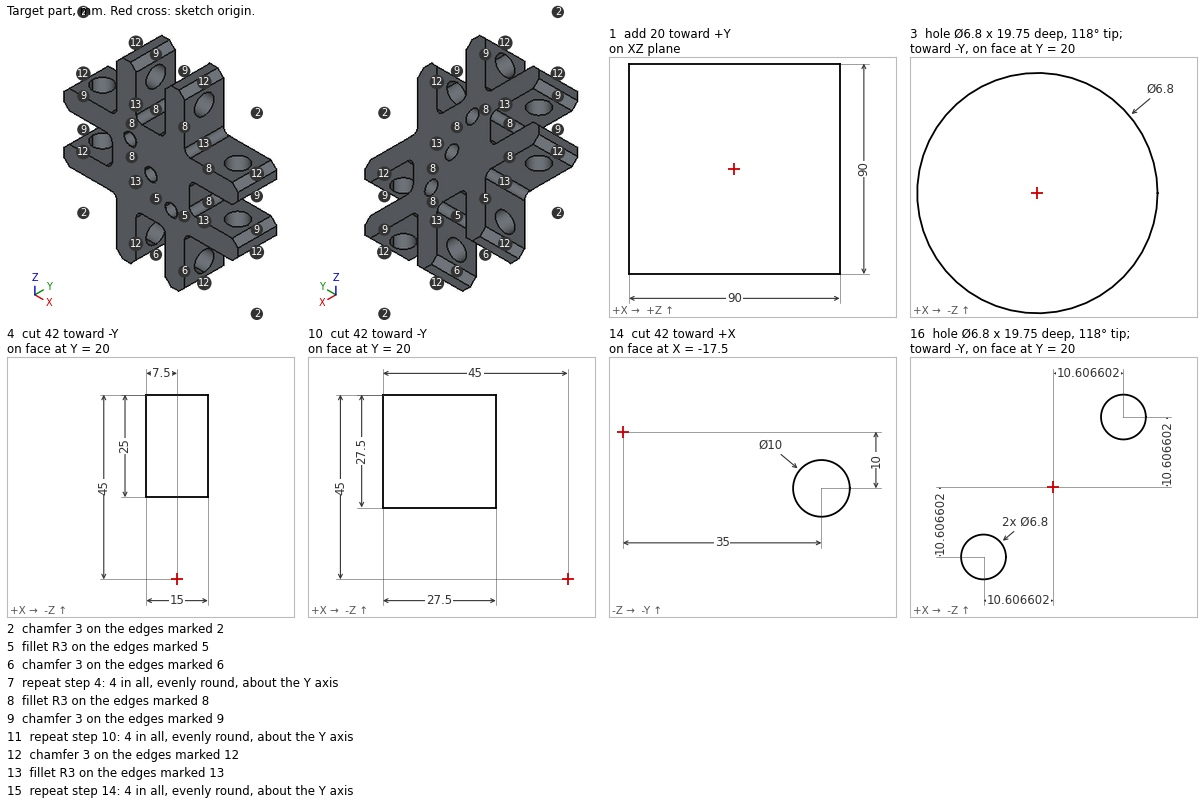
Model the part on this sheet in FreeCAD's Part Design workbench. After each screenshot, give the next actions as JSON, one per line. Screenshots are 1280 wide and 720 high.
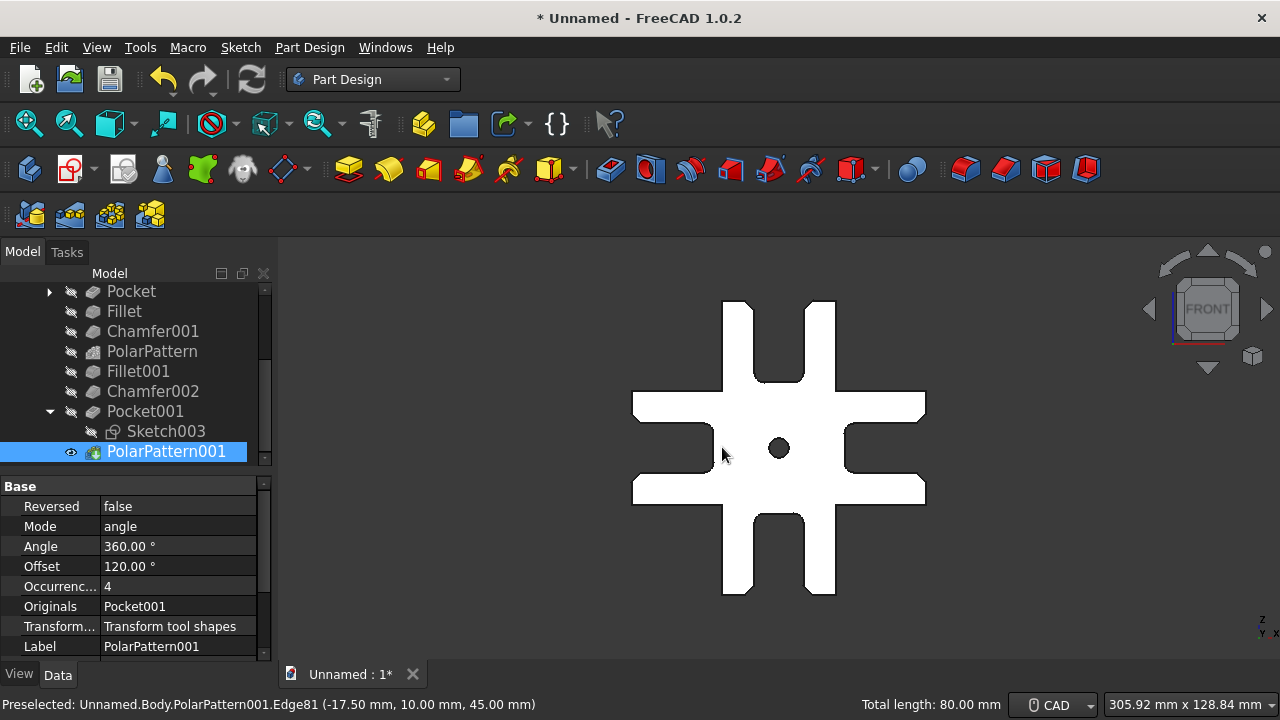
{"action": "key", "text": "3"}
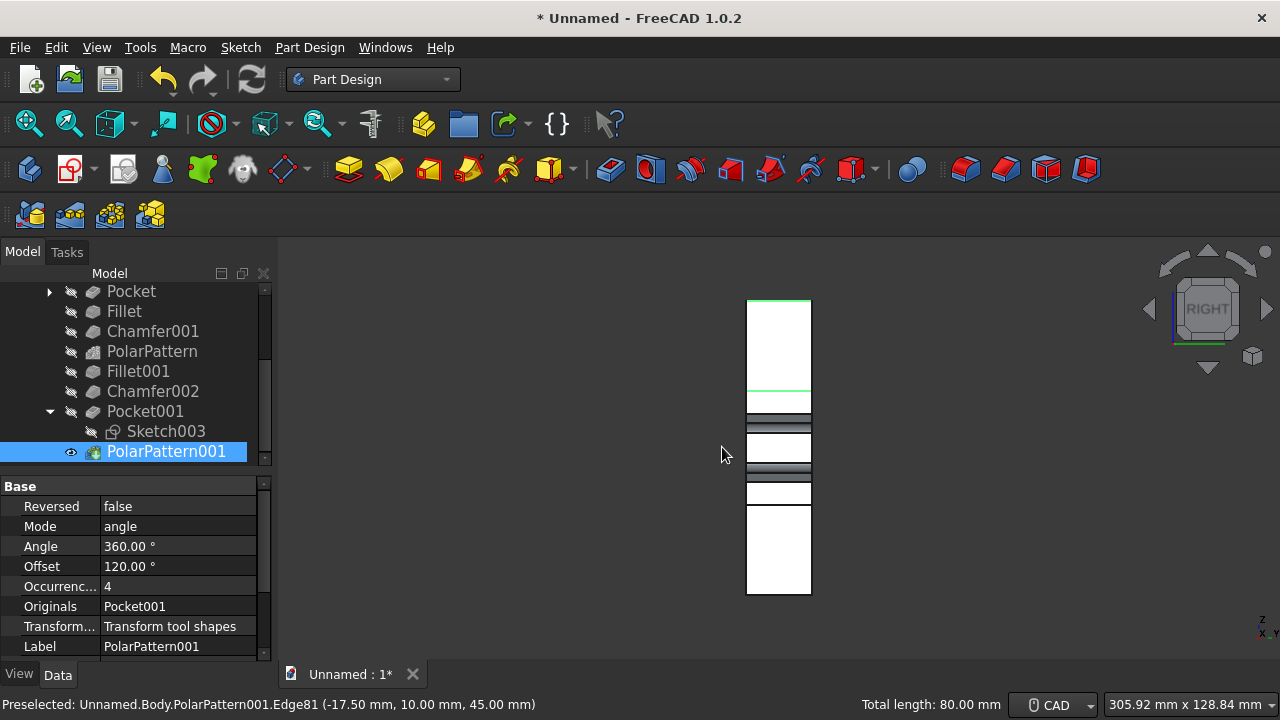
{"action": "left_click", "coordinate": [779, 504], "text": "ctrl"}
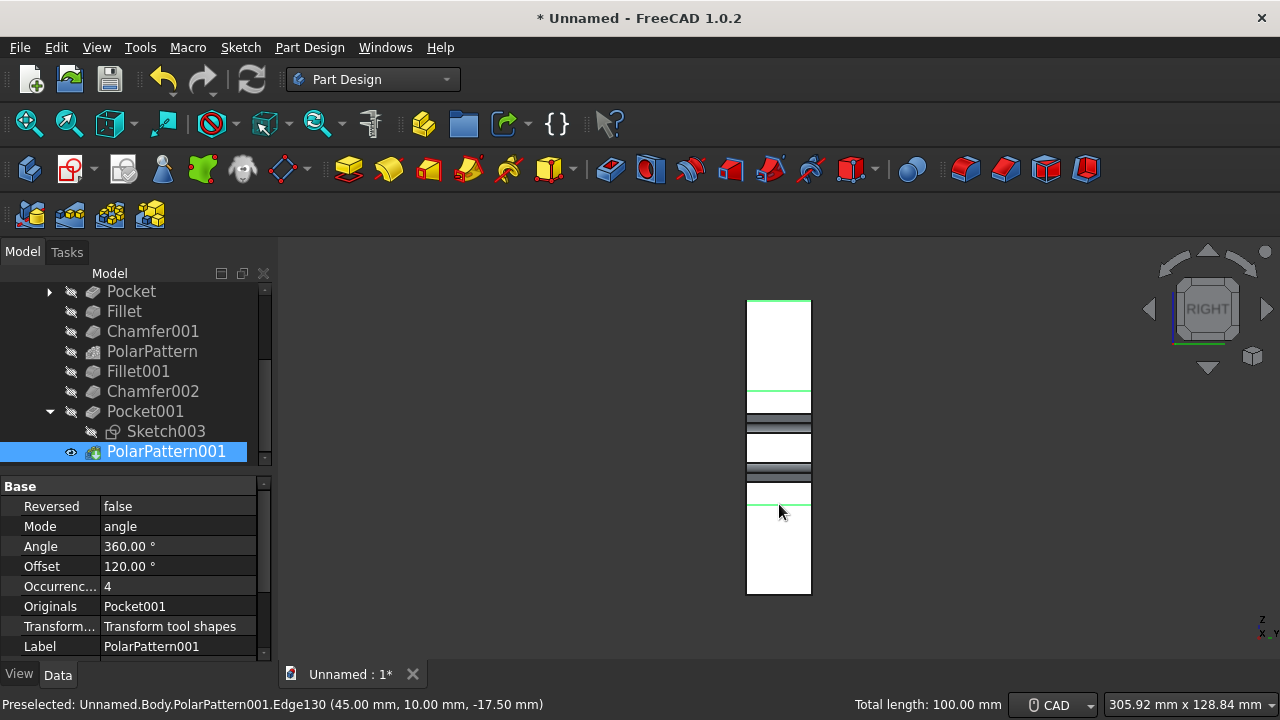
{"action": "left_click", "coordinate": [779, 594], "text": "ctrl"}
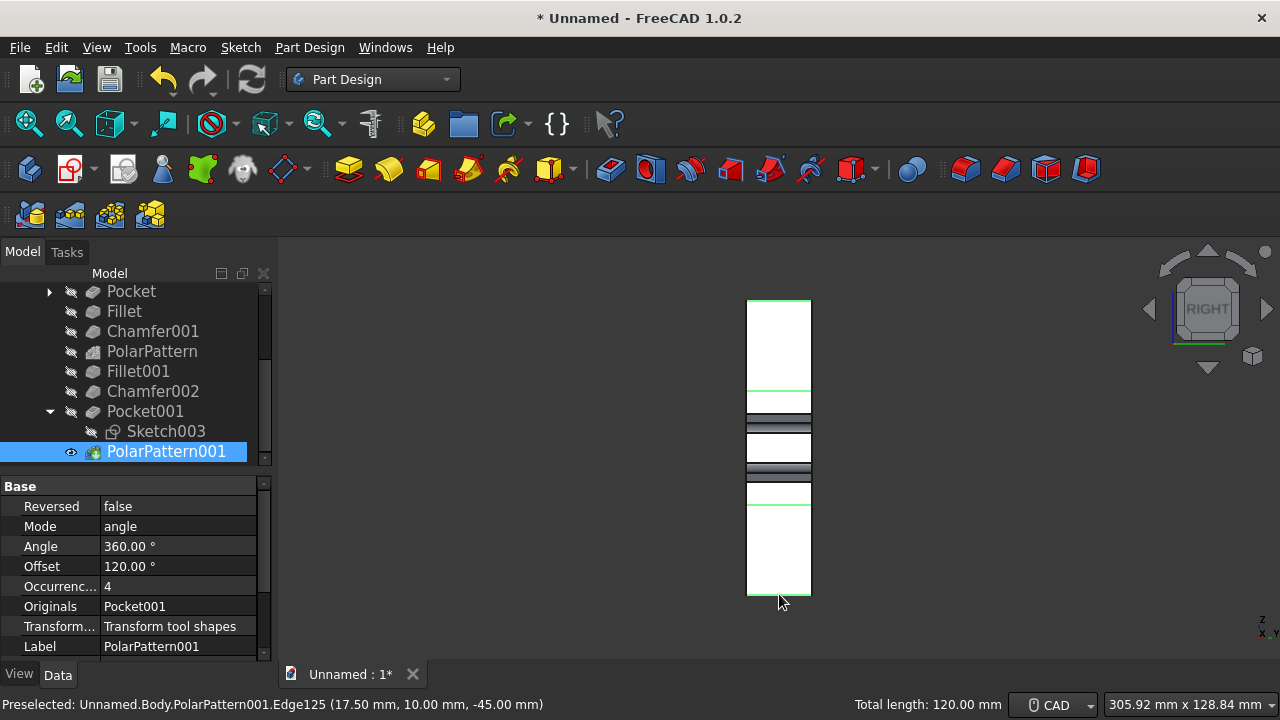
{"action": "key", "text": "5"}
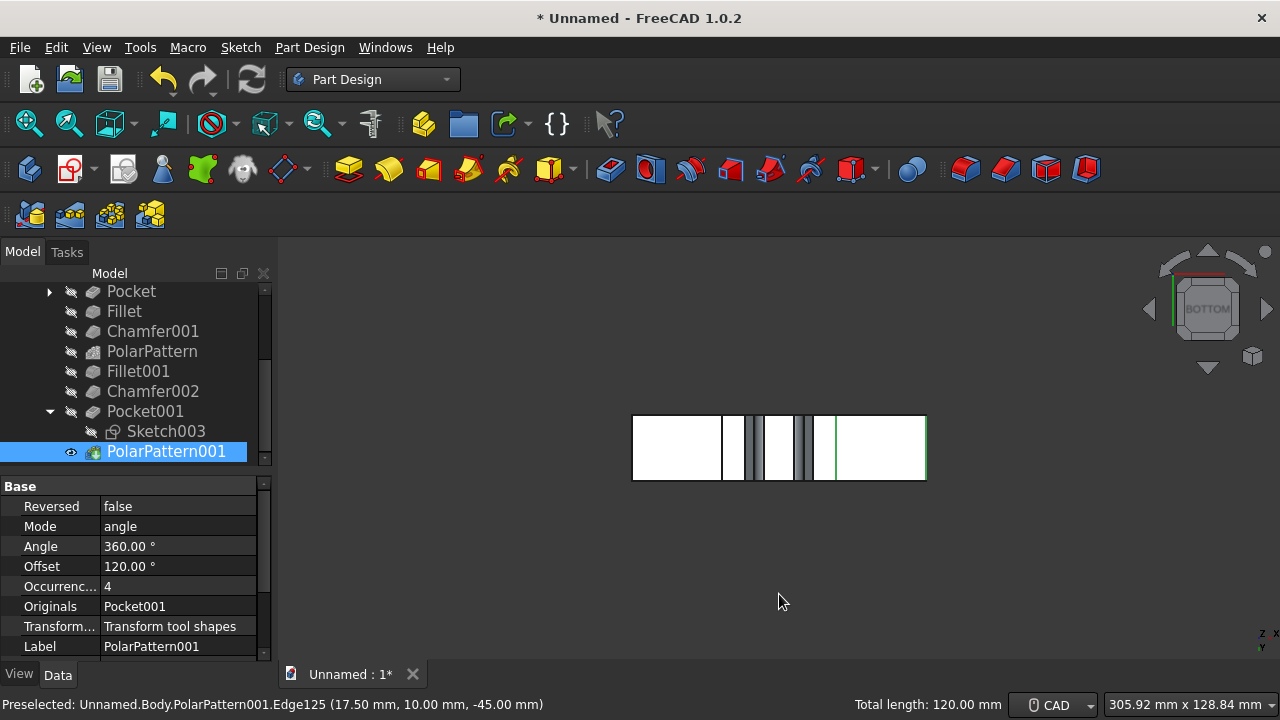
{"action": "left_click", "coordinate": [30, 124]}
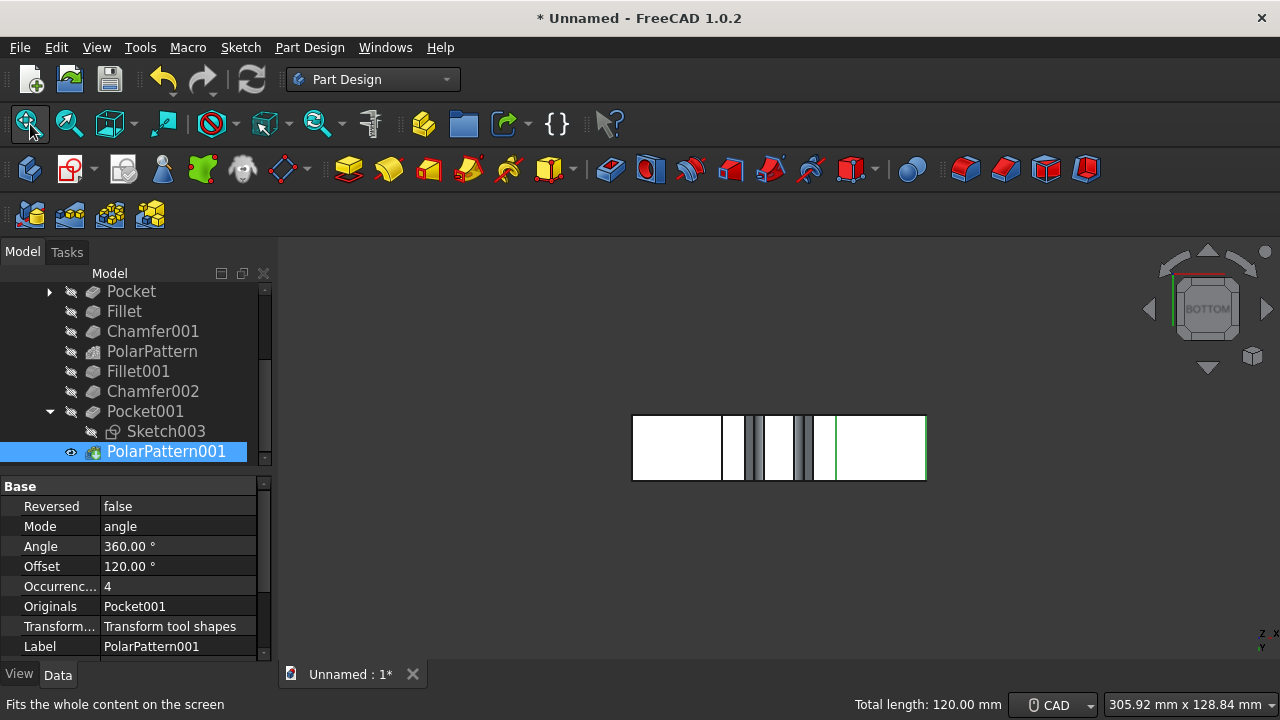
{"action": "left_click", "coordinate": [722, 447], "text": "ctrl"}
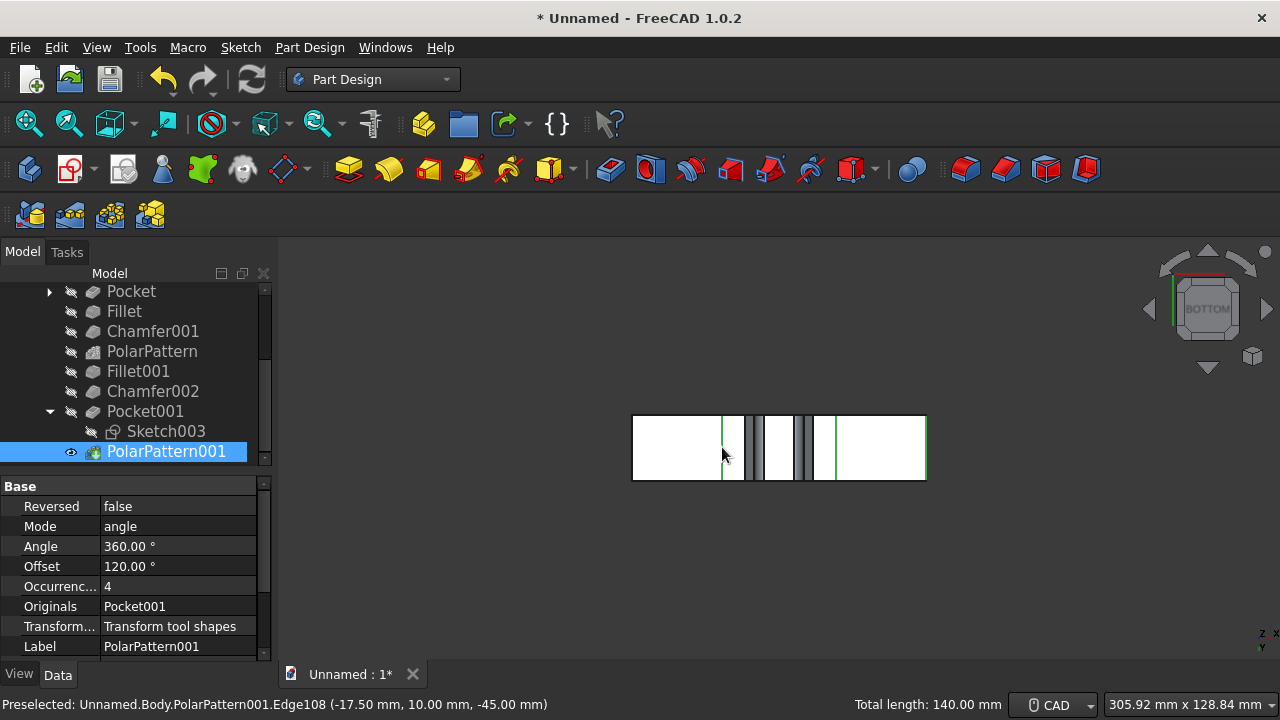
{"action": "left_click", "coordinate": [632, 447], "text": "ctrl"}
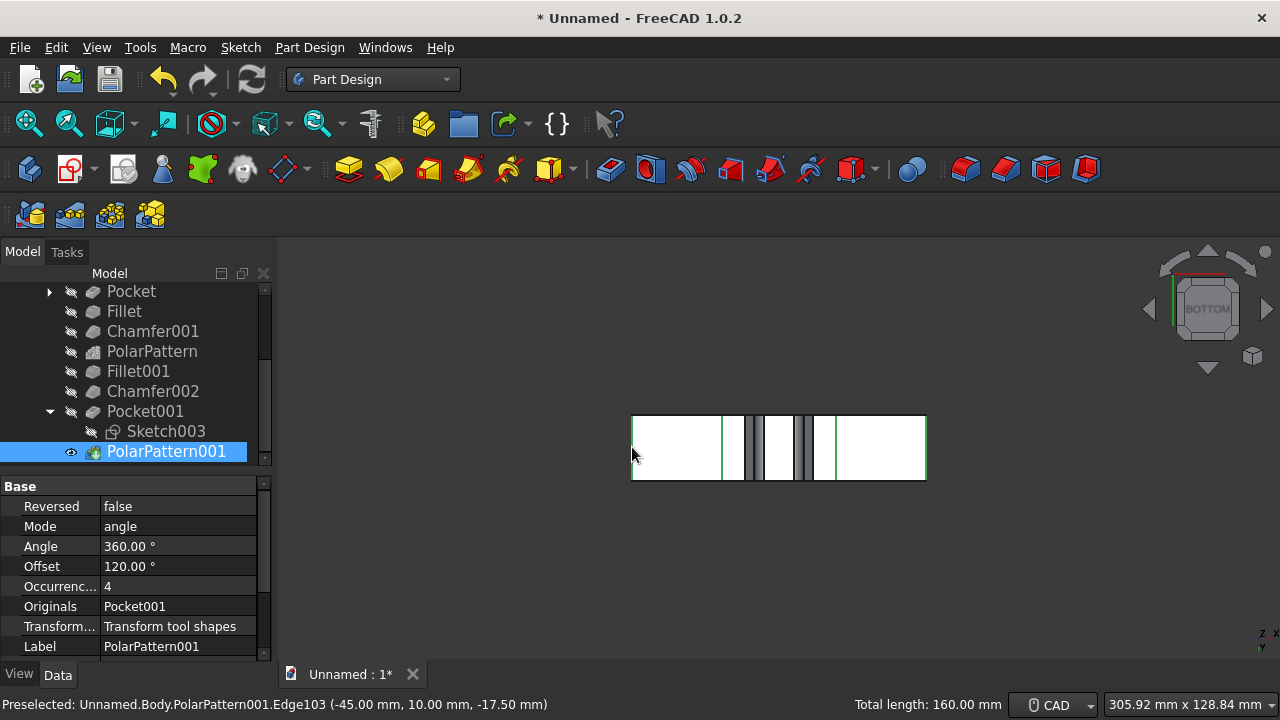
{"action": "left_click", "coordinate": [1006, 170]}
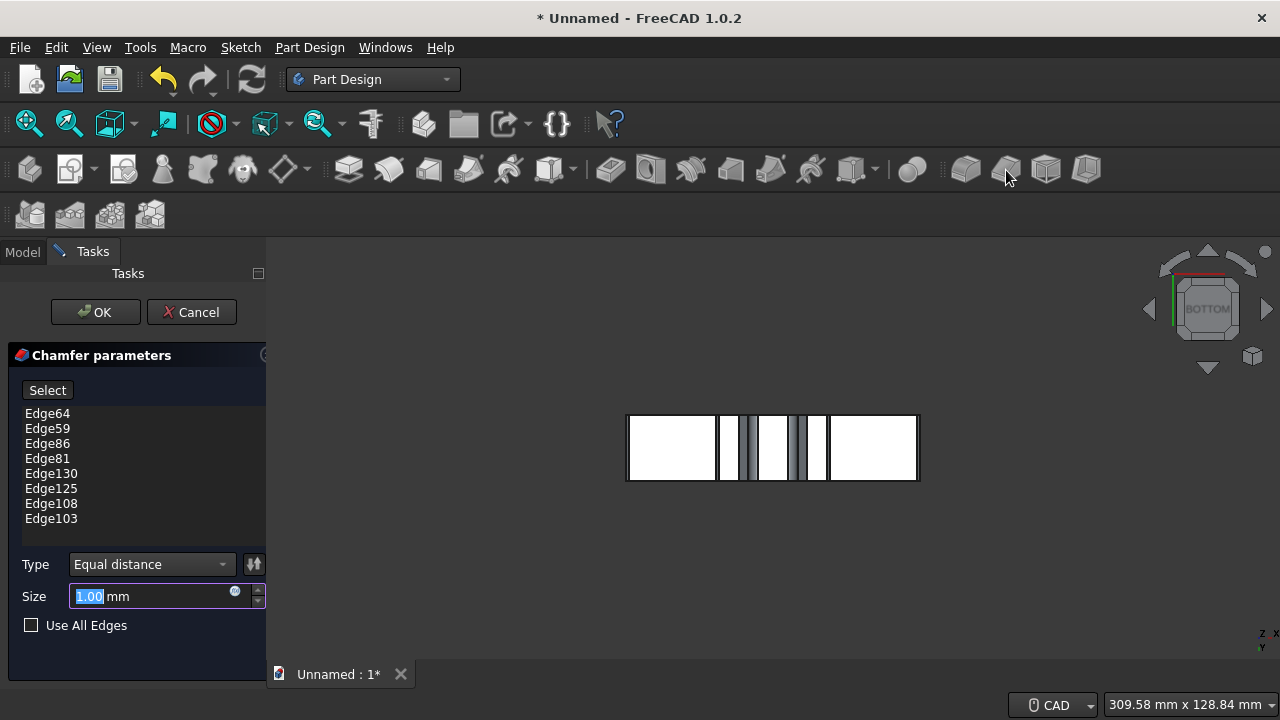
{"action": "type", "text": "3"}
{"action": "key", "text": "Tab"}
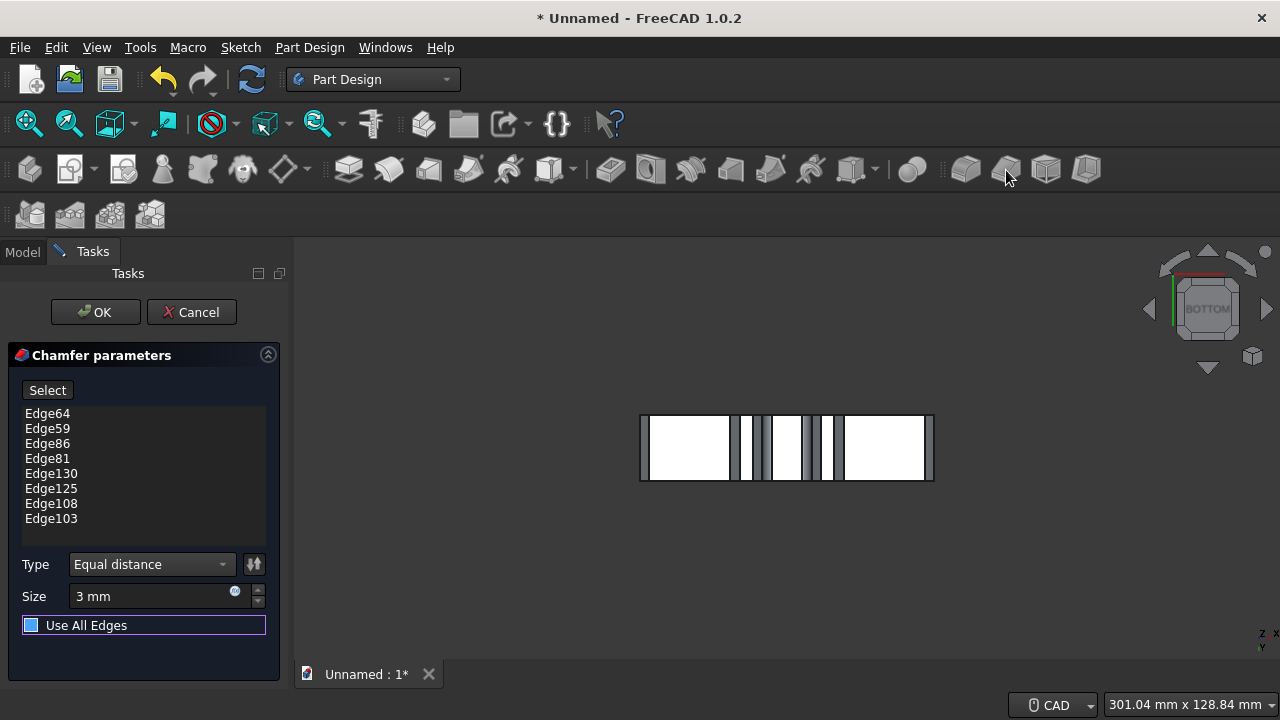
{"action": "left_click", "coordinate": [96, 312]}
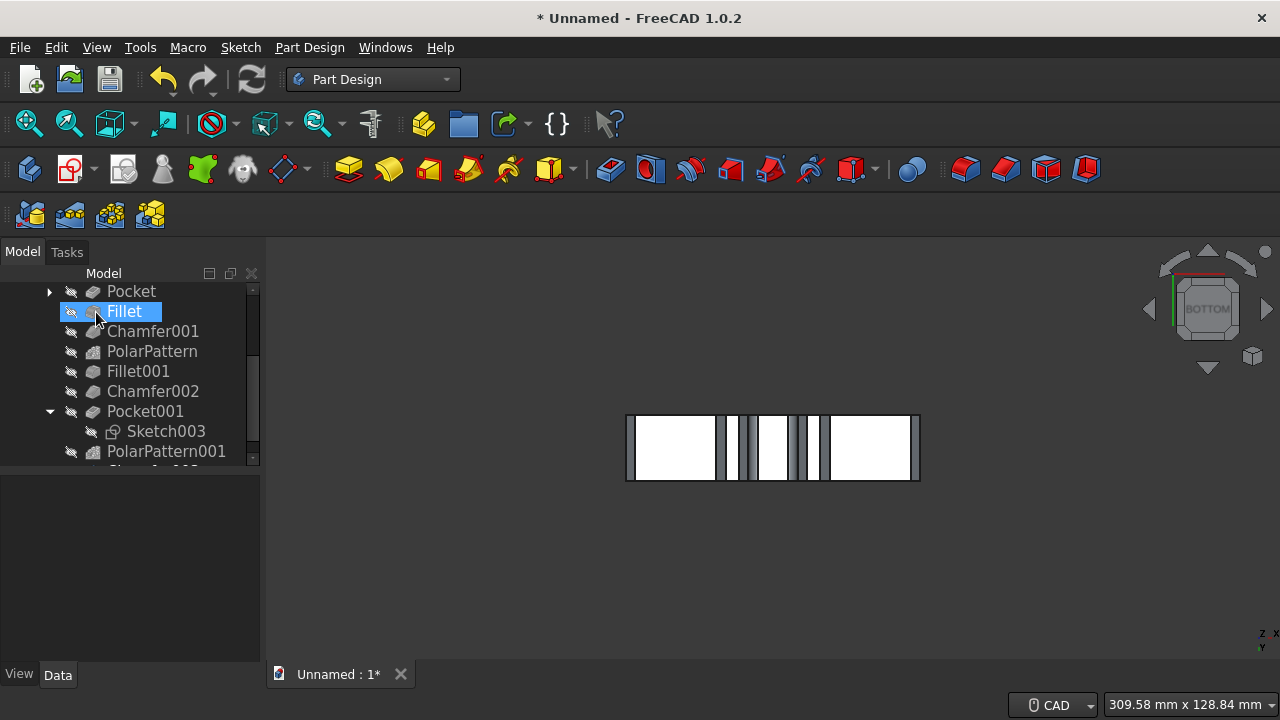
{"action": "left_click", "coordinate": [30, 124]}